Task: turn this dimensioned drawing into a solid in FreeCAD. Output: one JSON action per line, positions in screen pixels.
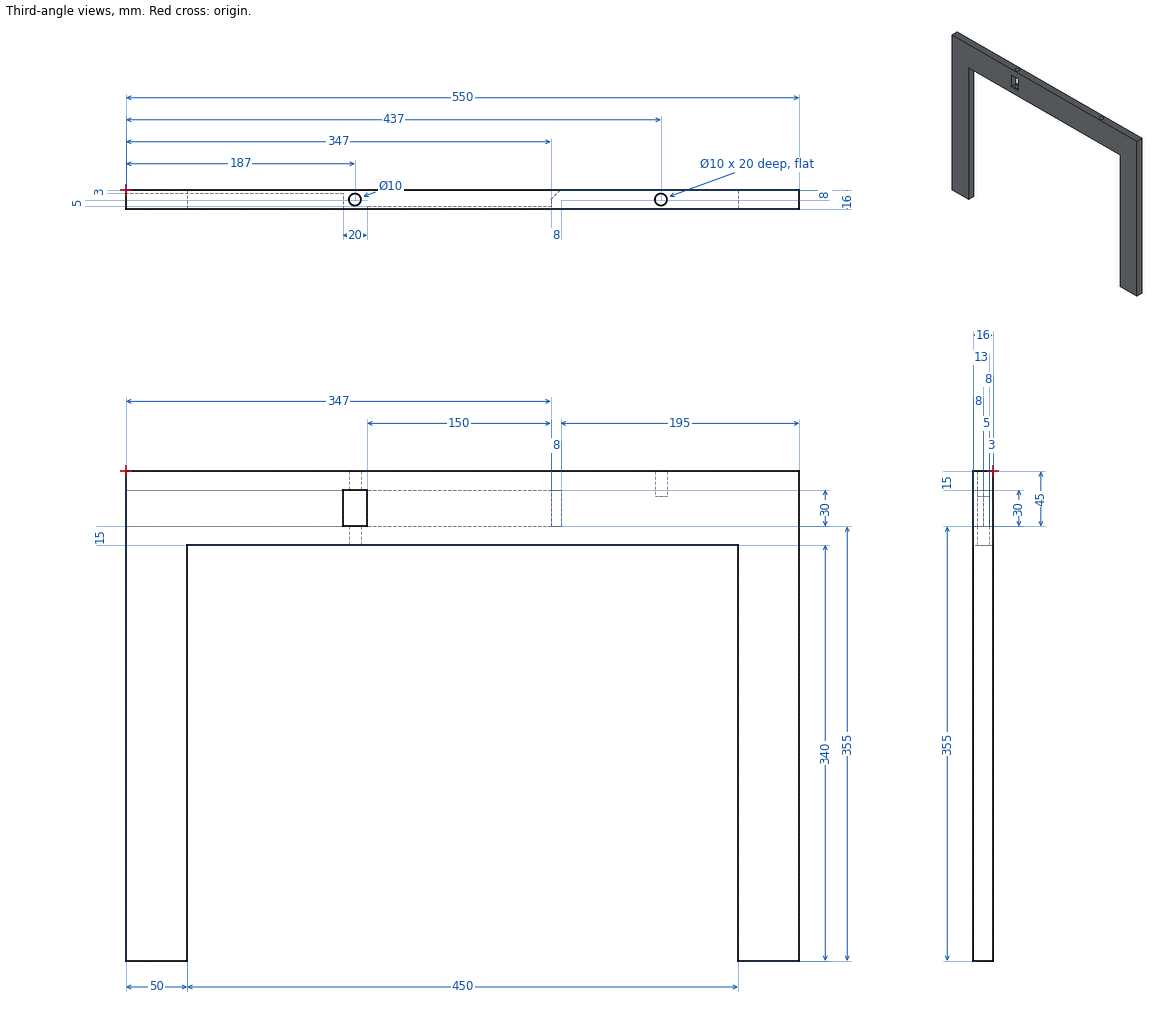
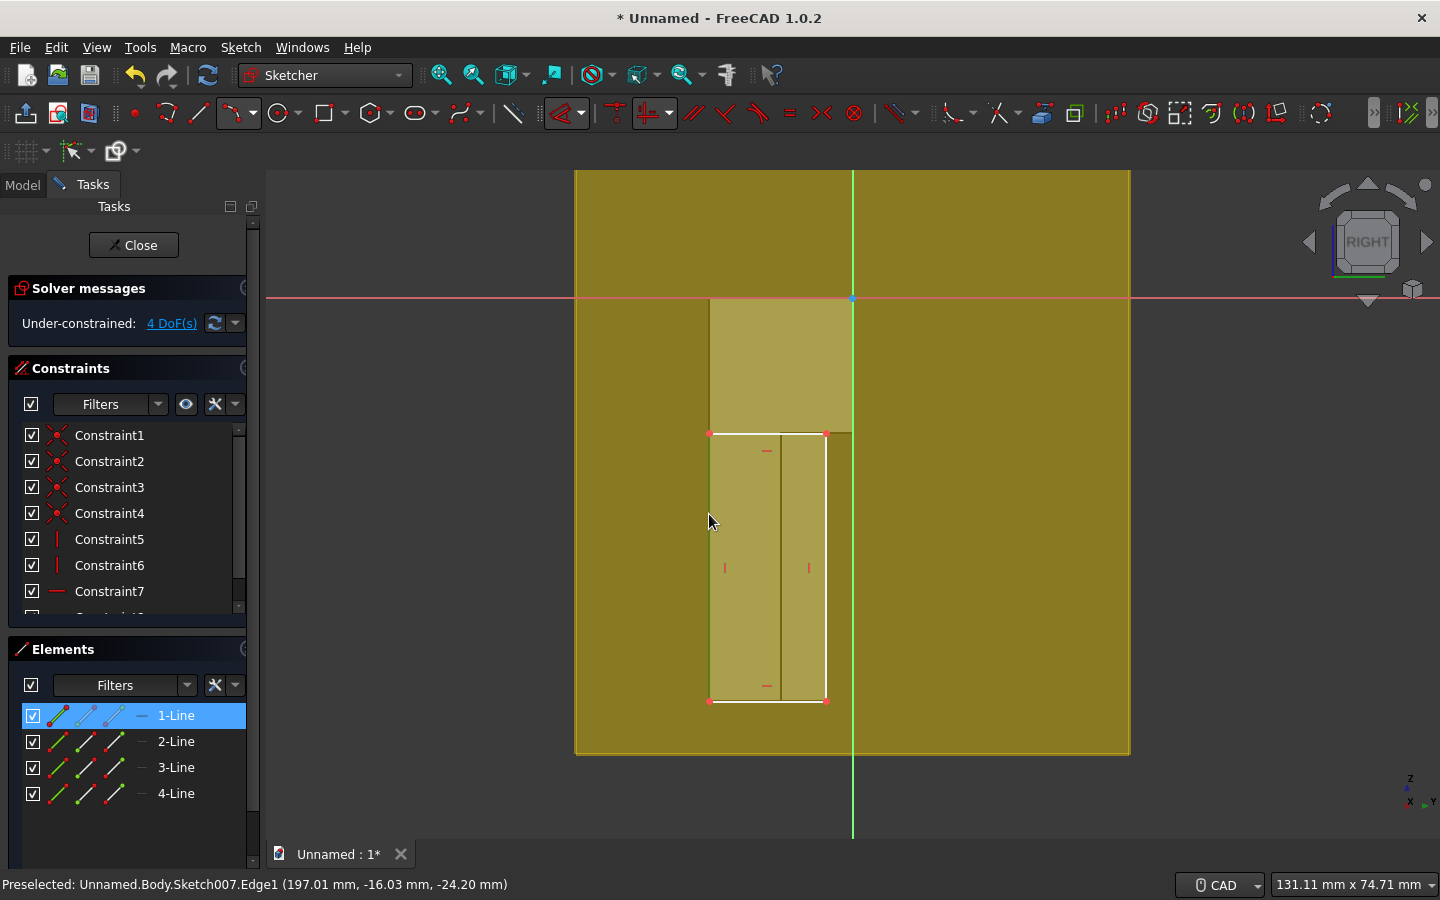
{"action": "key", "text": "i"}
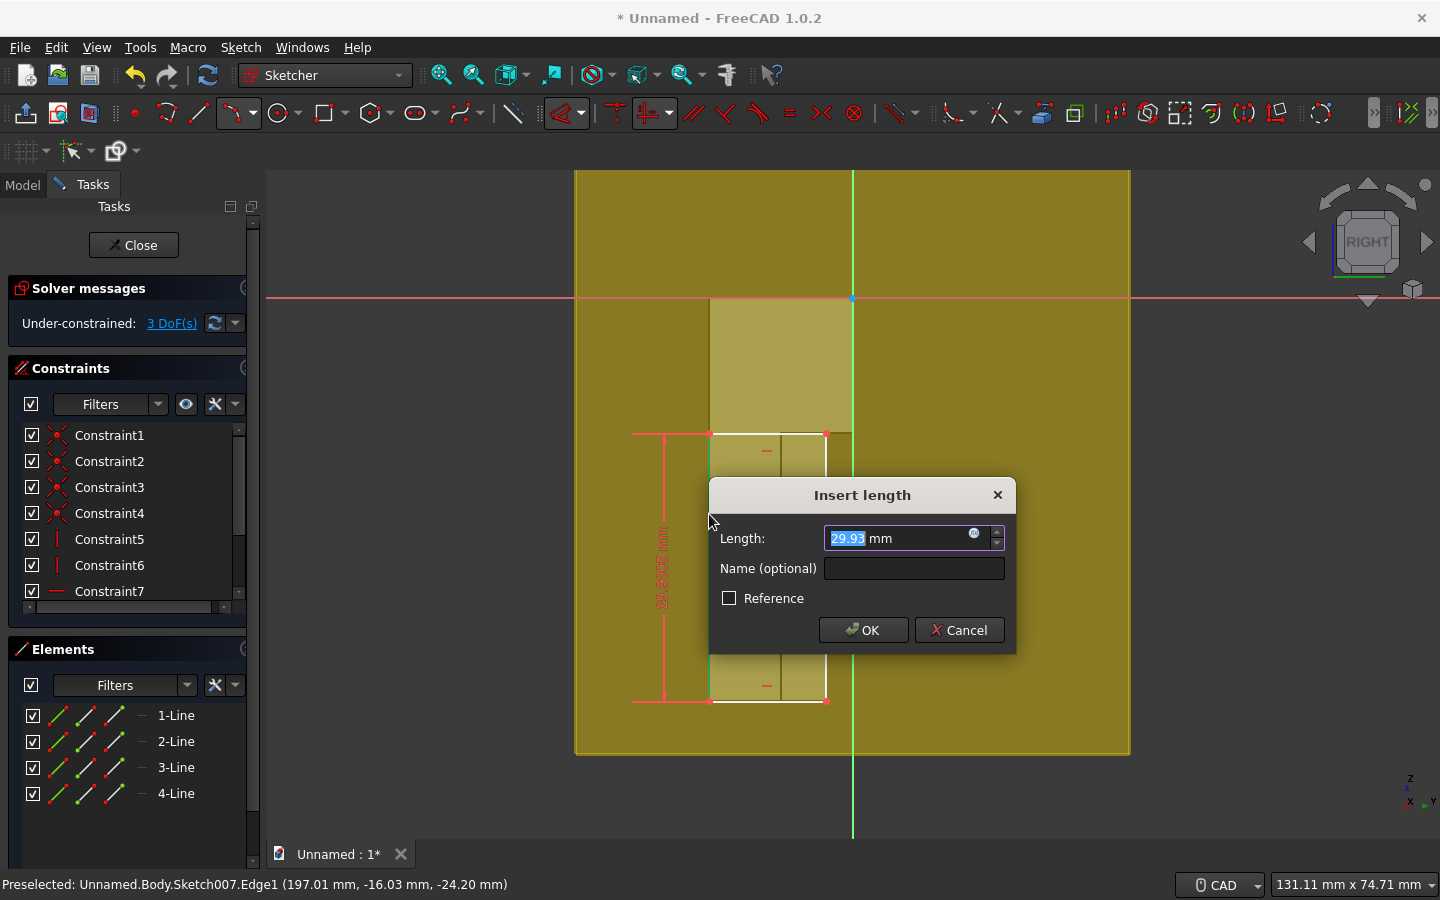
{"action": "type", "text": "30"}
{"action": "key", "text": "Return"}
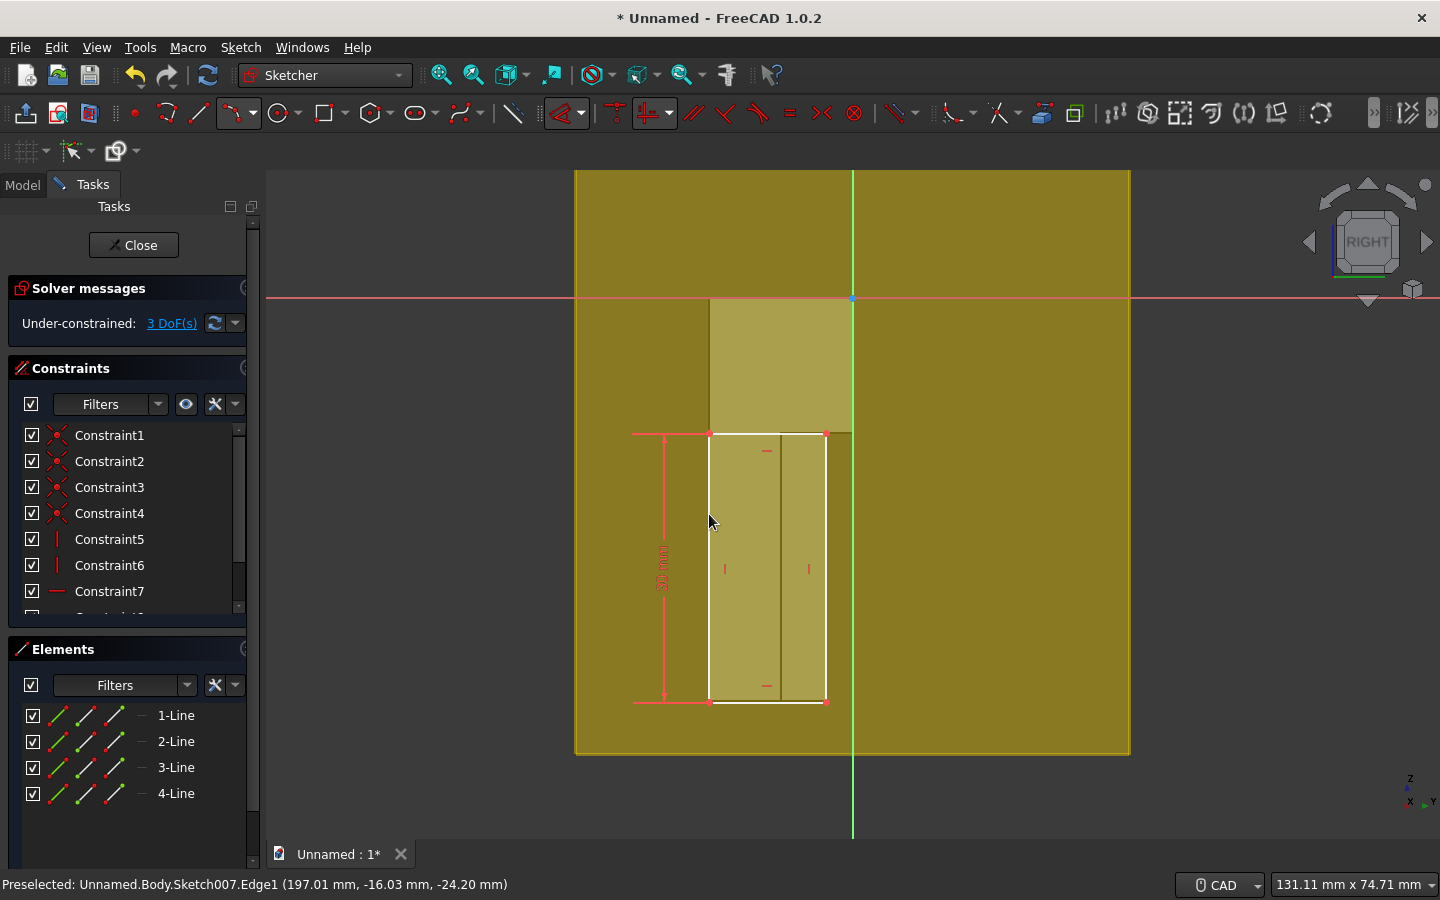
{"action": "left_click", "coordinate": [744, 703]}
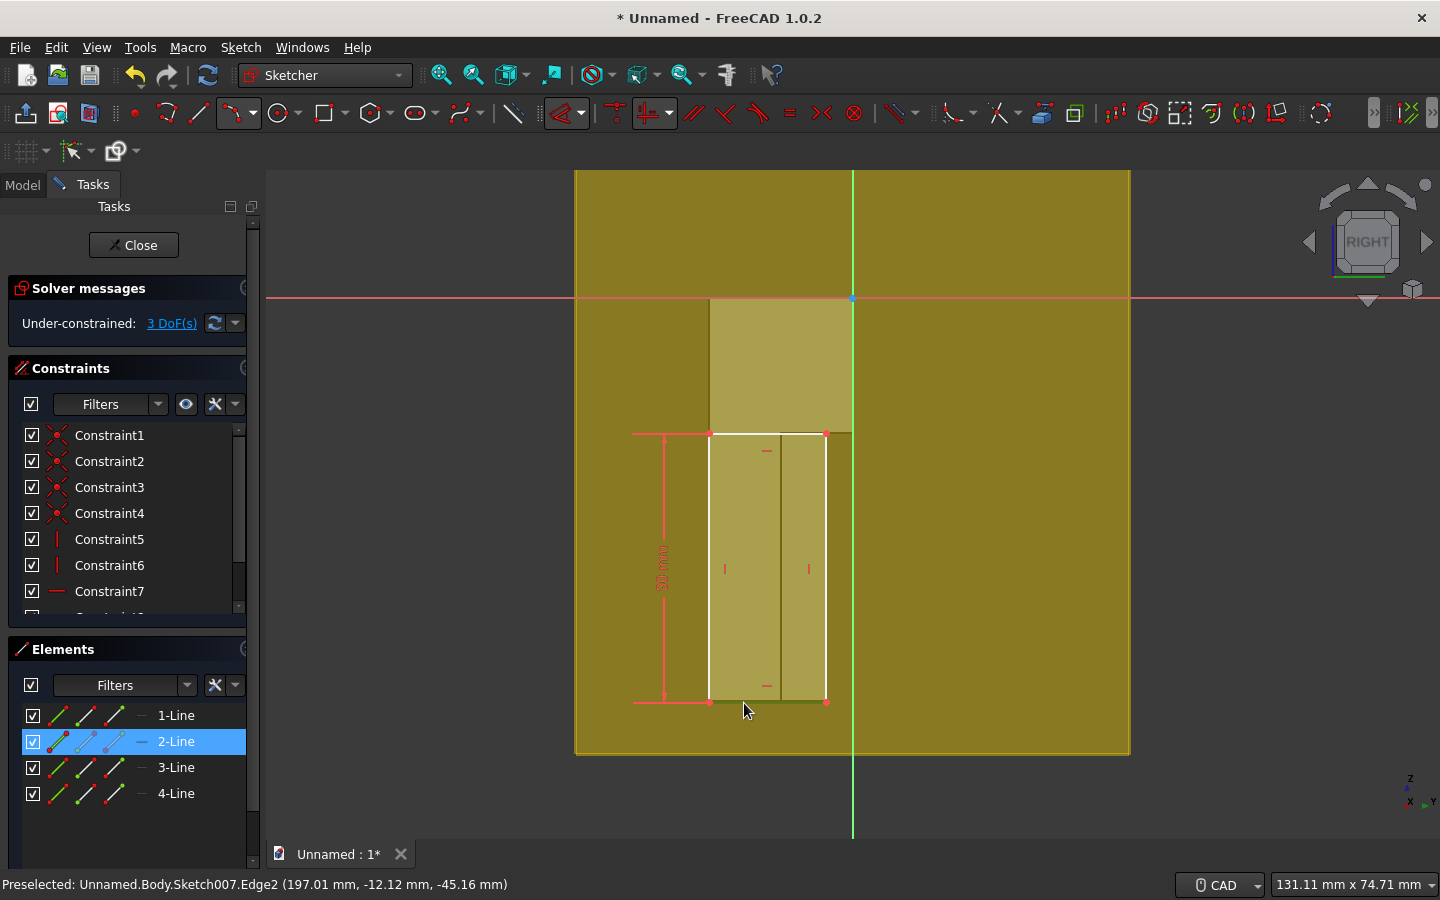
{"action": "left_click", "coordinate": [584, 114]}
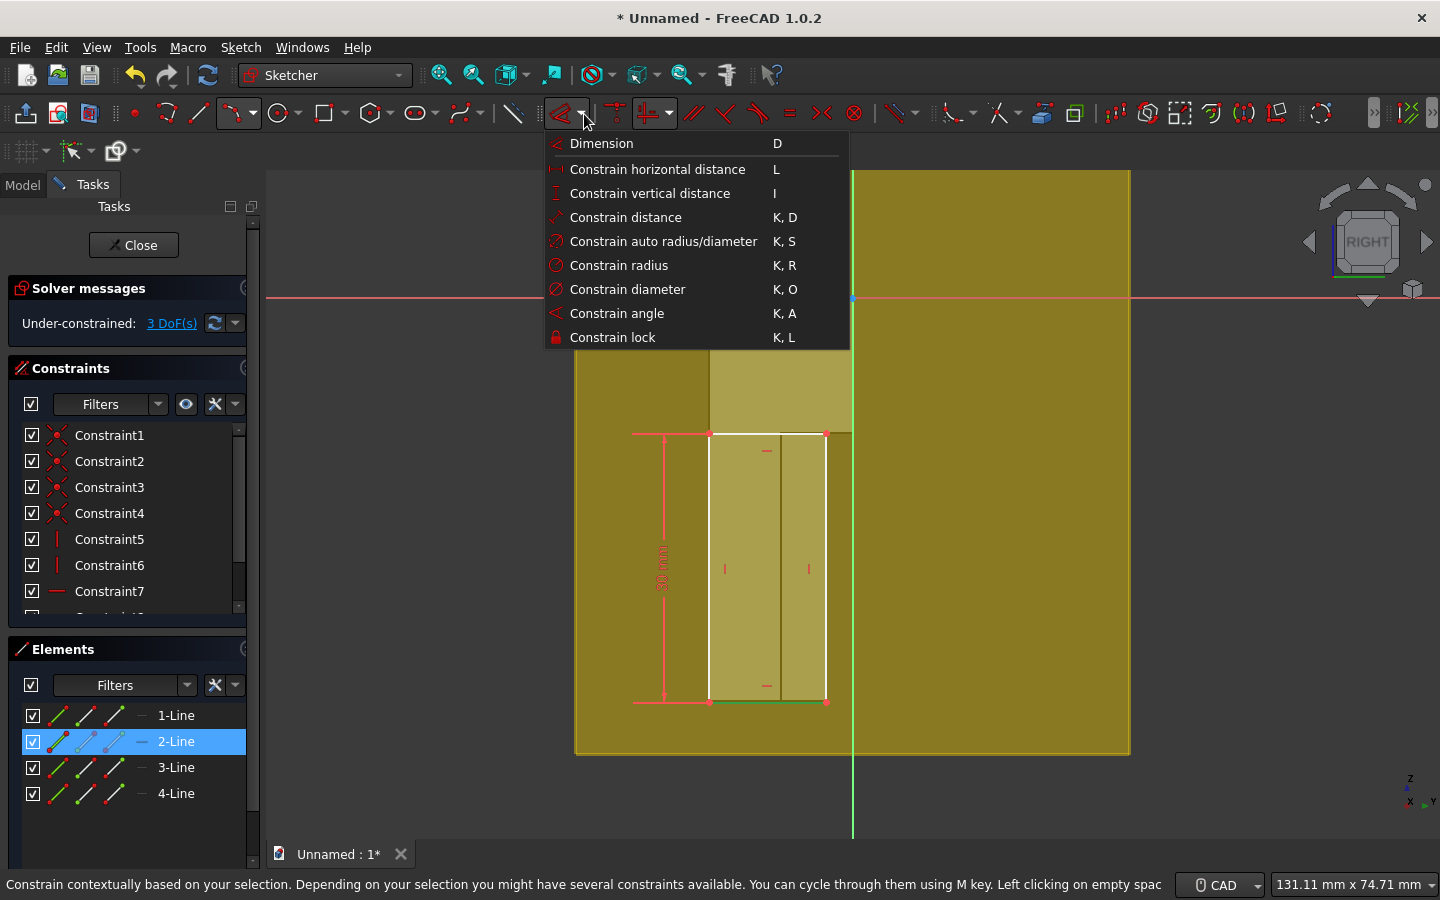
{"action": "left_click", "coordinate": [697, 169]}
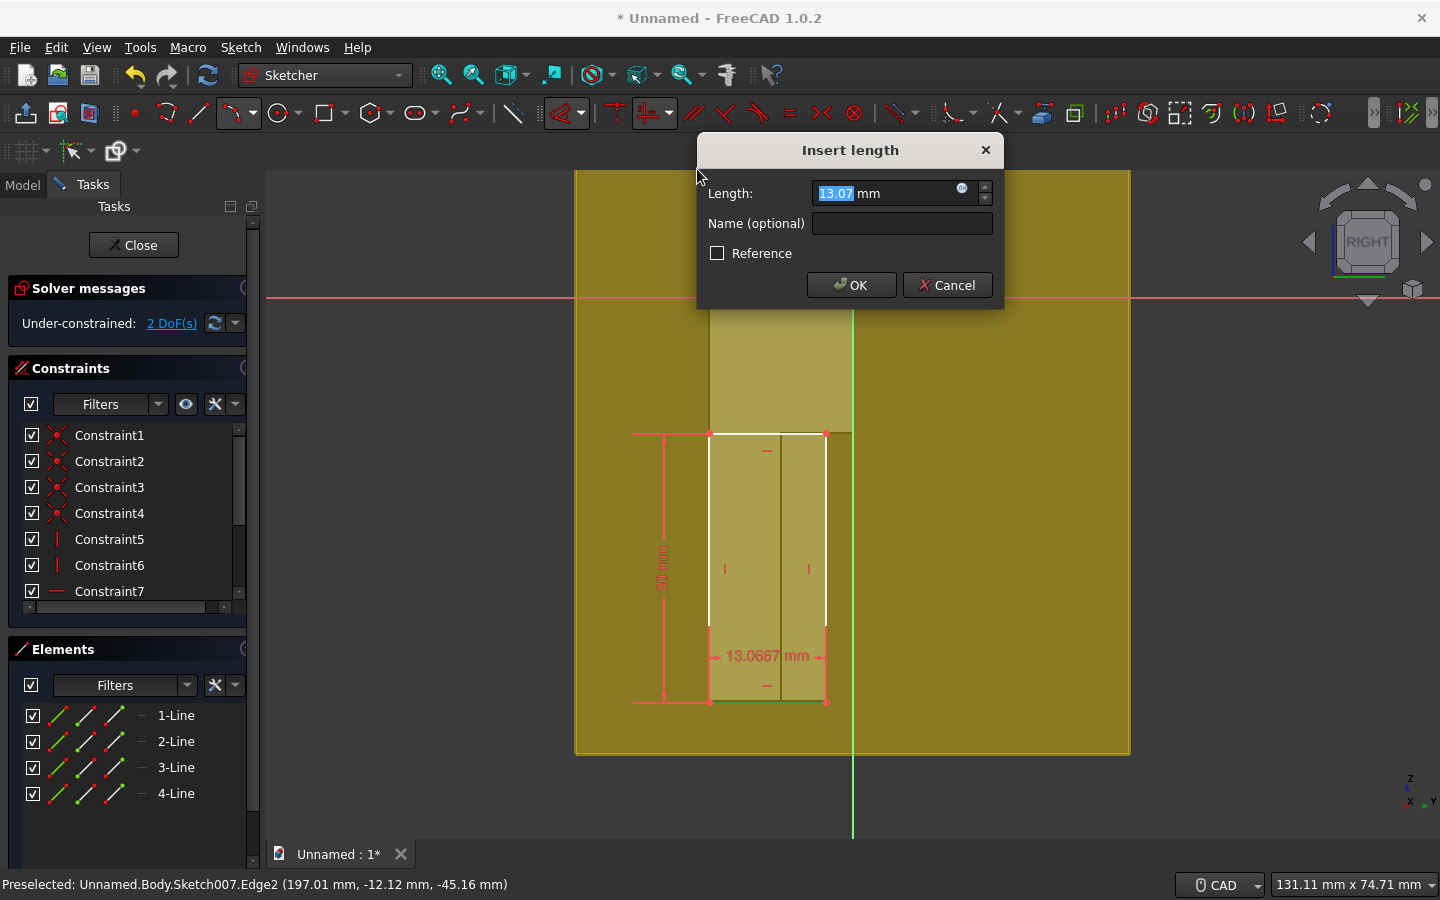
{"action": "type", "text": "13"}
{"action": "key", "text": "Return"}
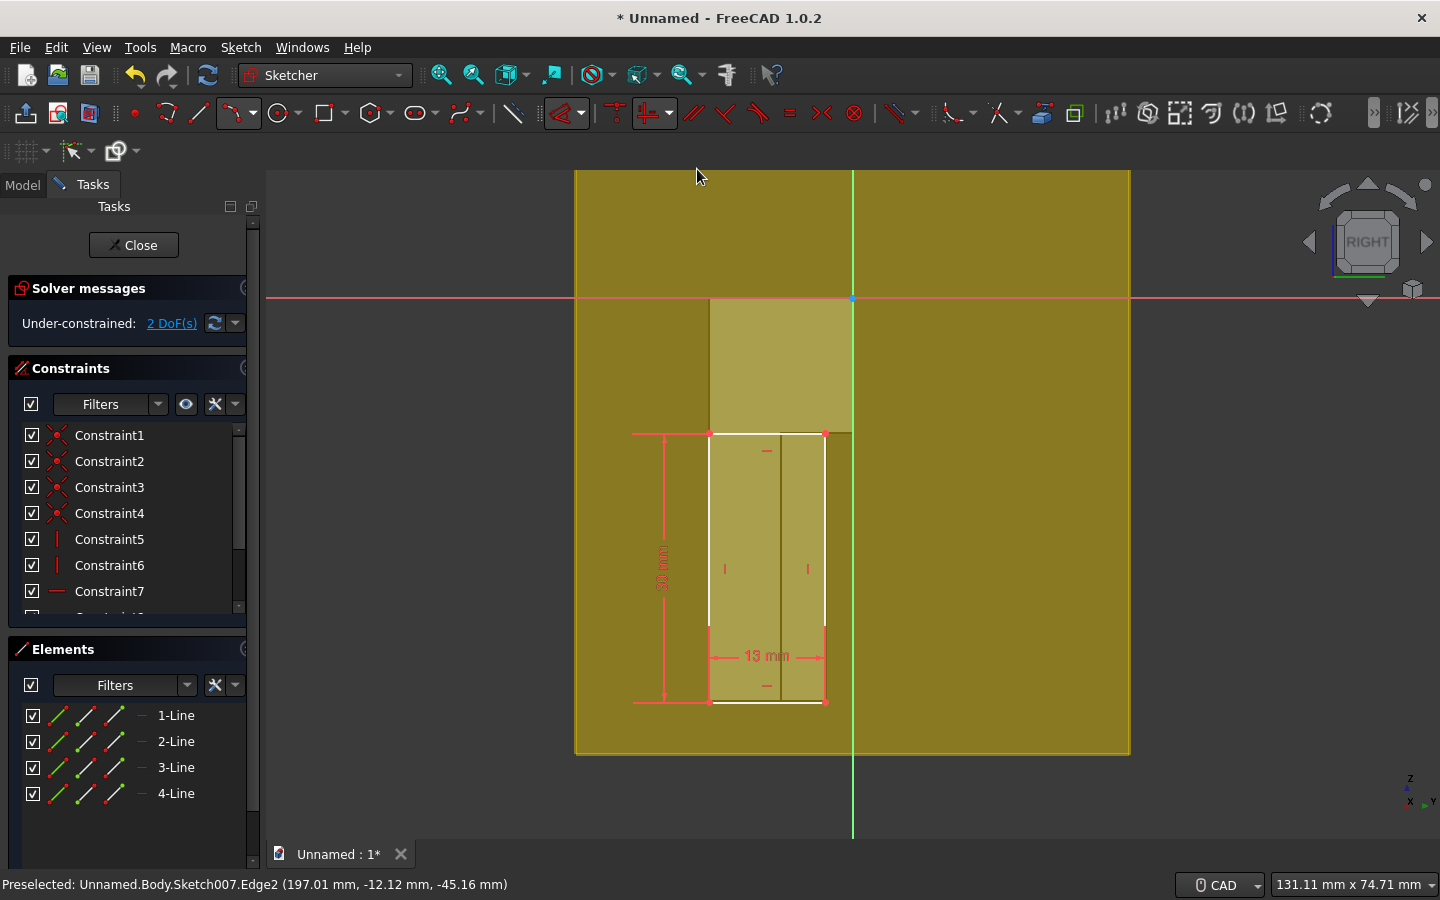
{"action": "scroll", "coordinate": [825, 703], "scroll_direction": "up", "scroll_amount": 2}